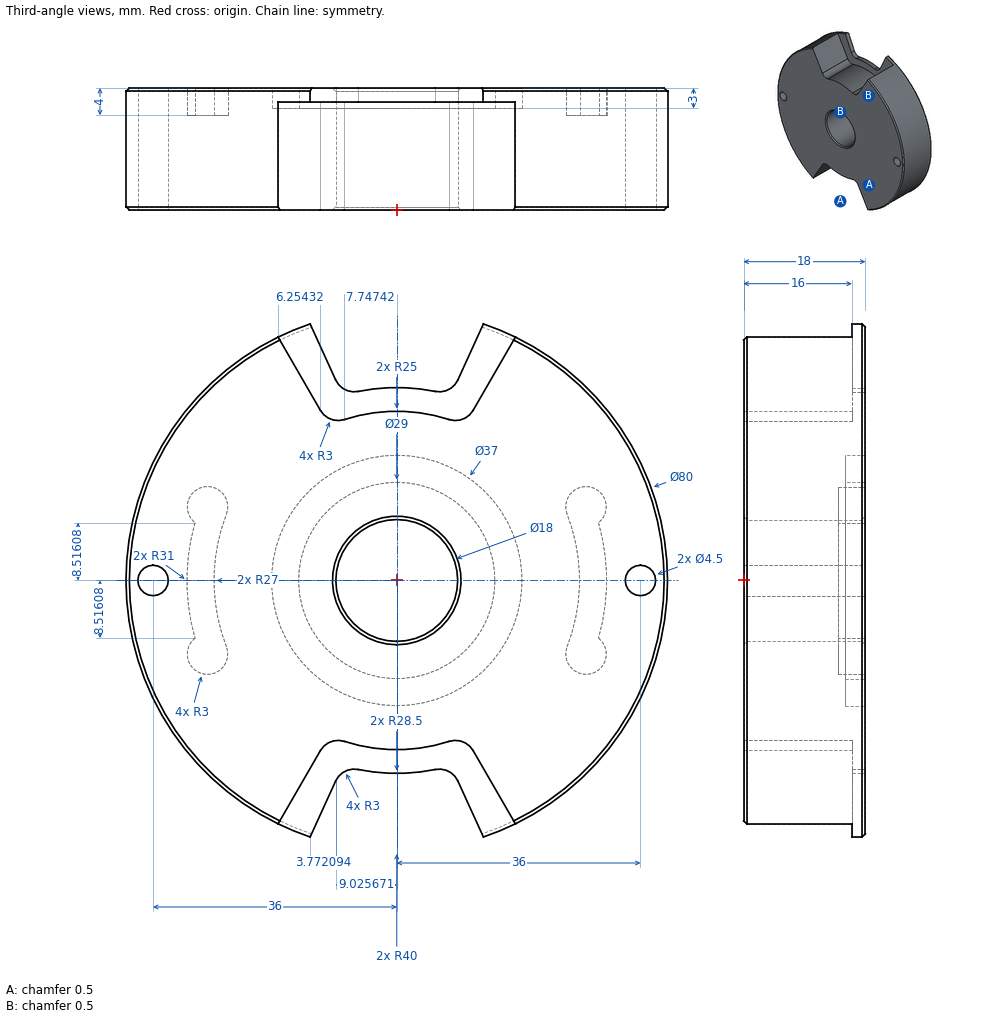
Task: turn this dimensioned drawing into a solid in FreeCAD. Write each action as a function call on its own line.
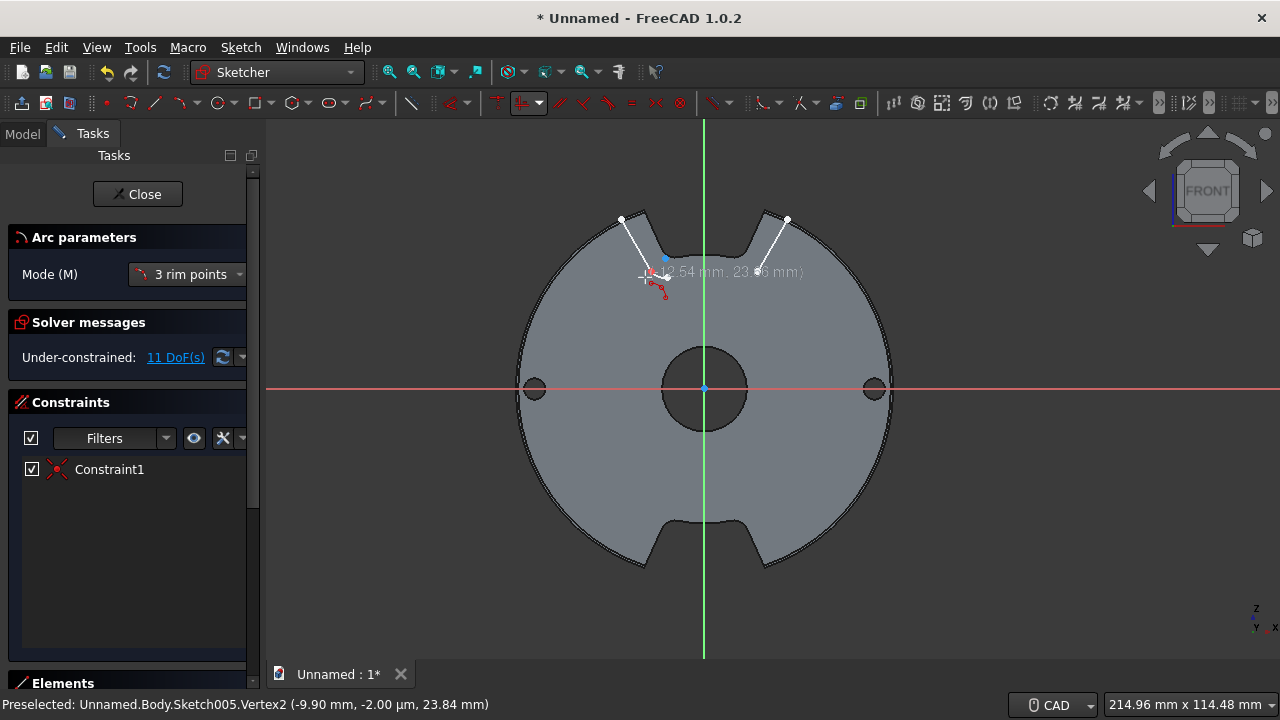
click(667, 278)
click(741, 277)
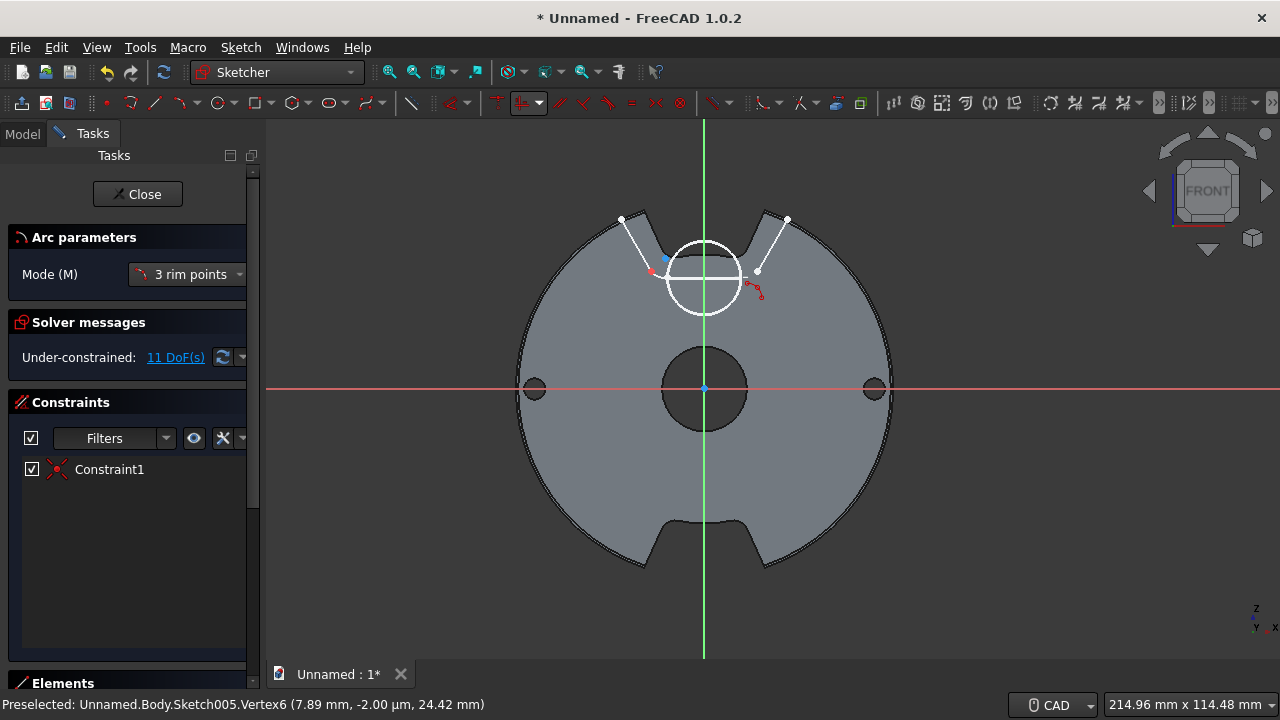
scroll(712, 271, up, 6)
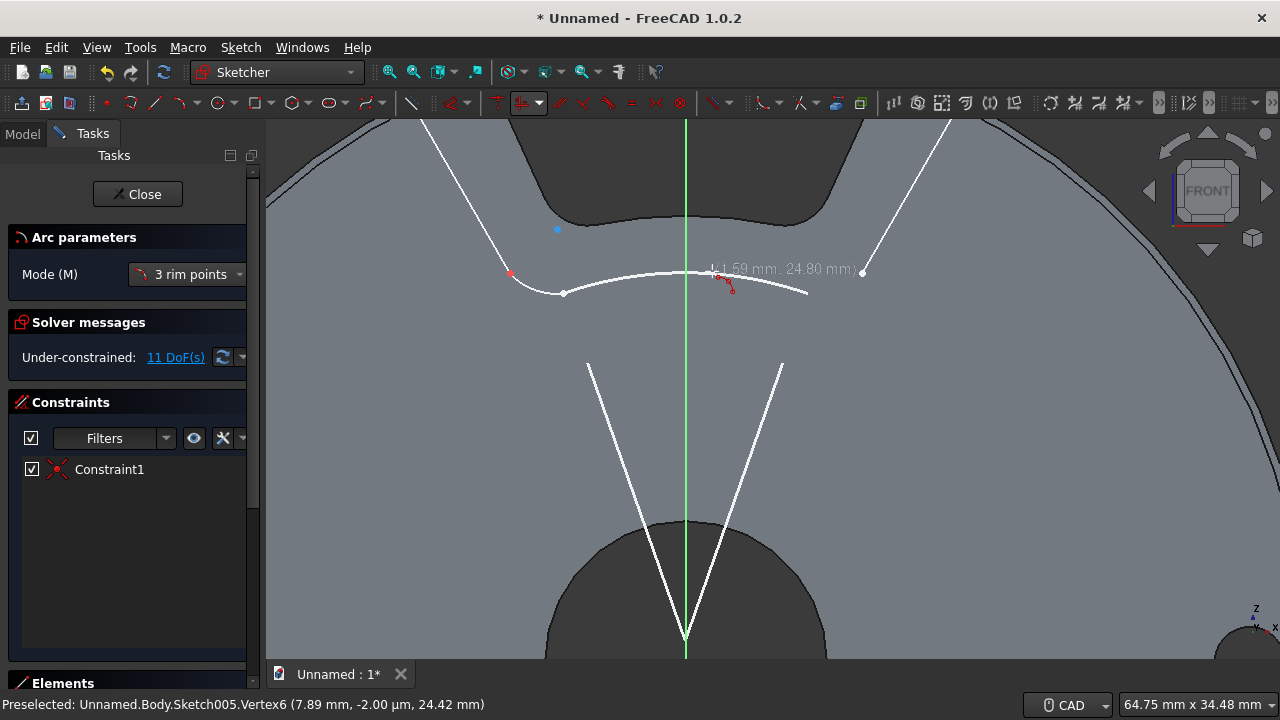
click(711, 271)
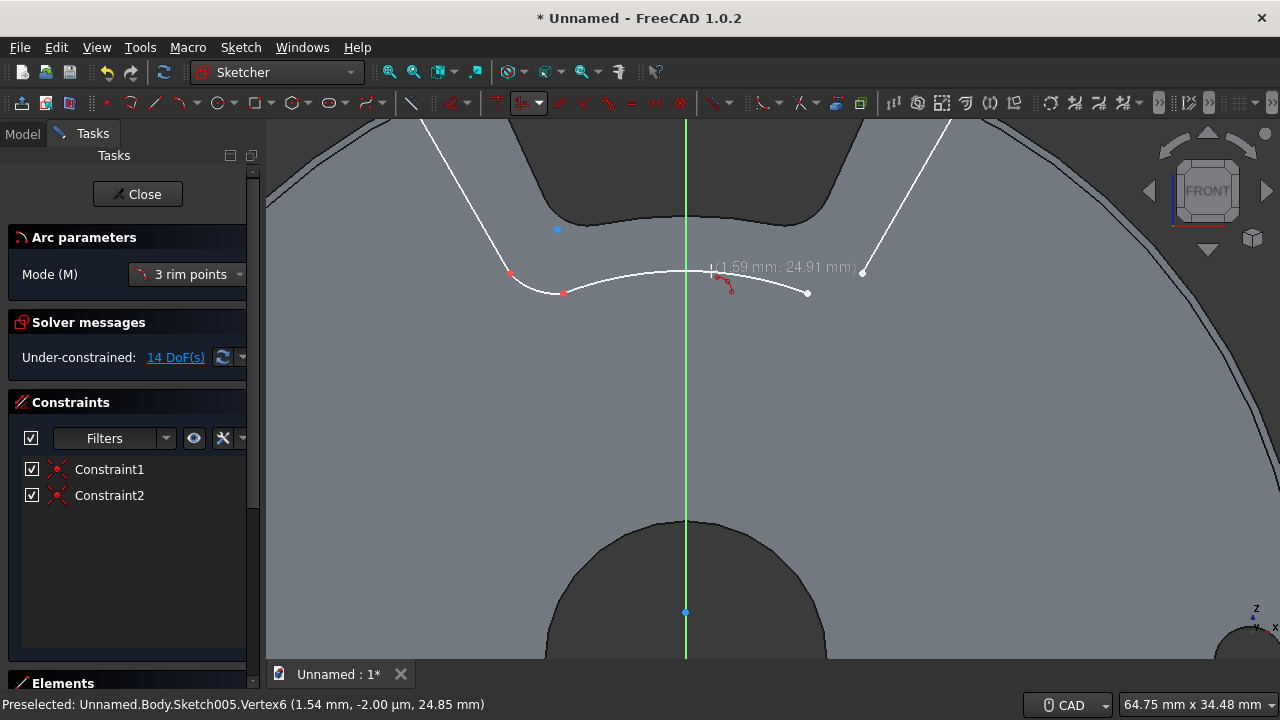
click(807, 294)
click(862, 274)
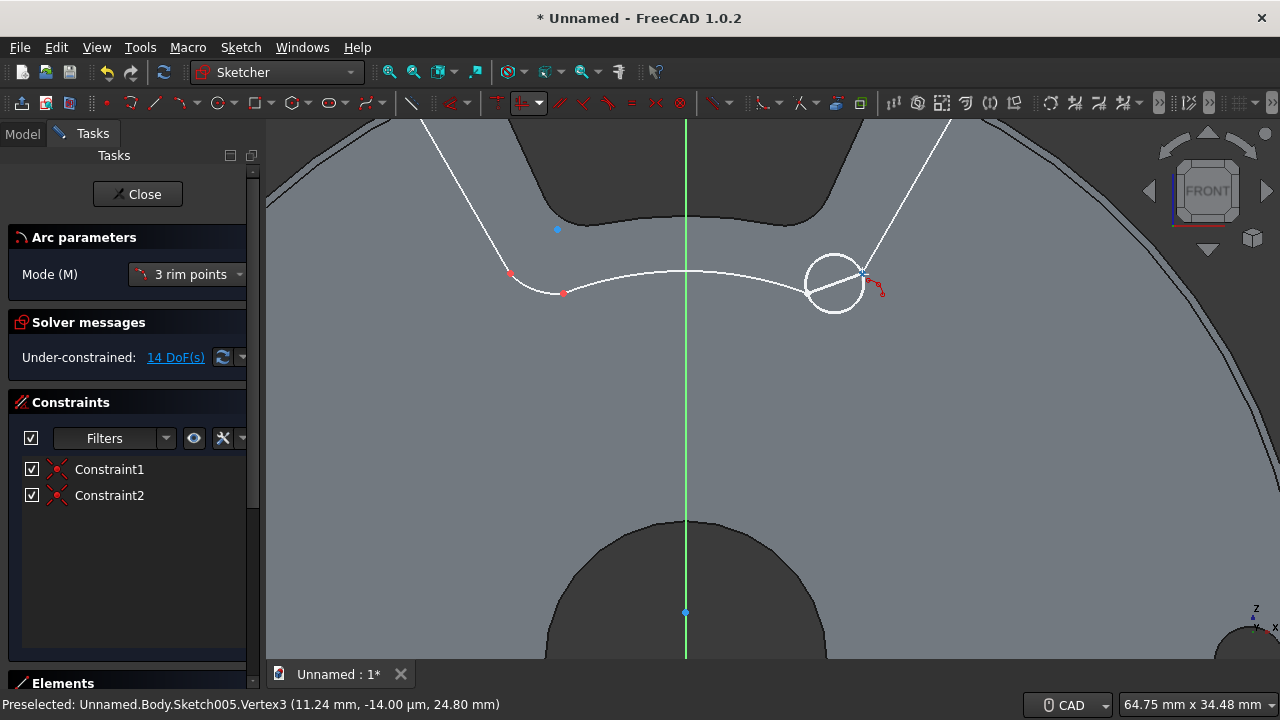
scroll(839, 289, up, 3)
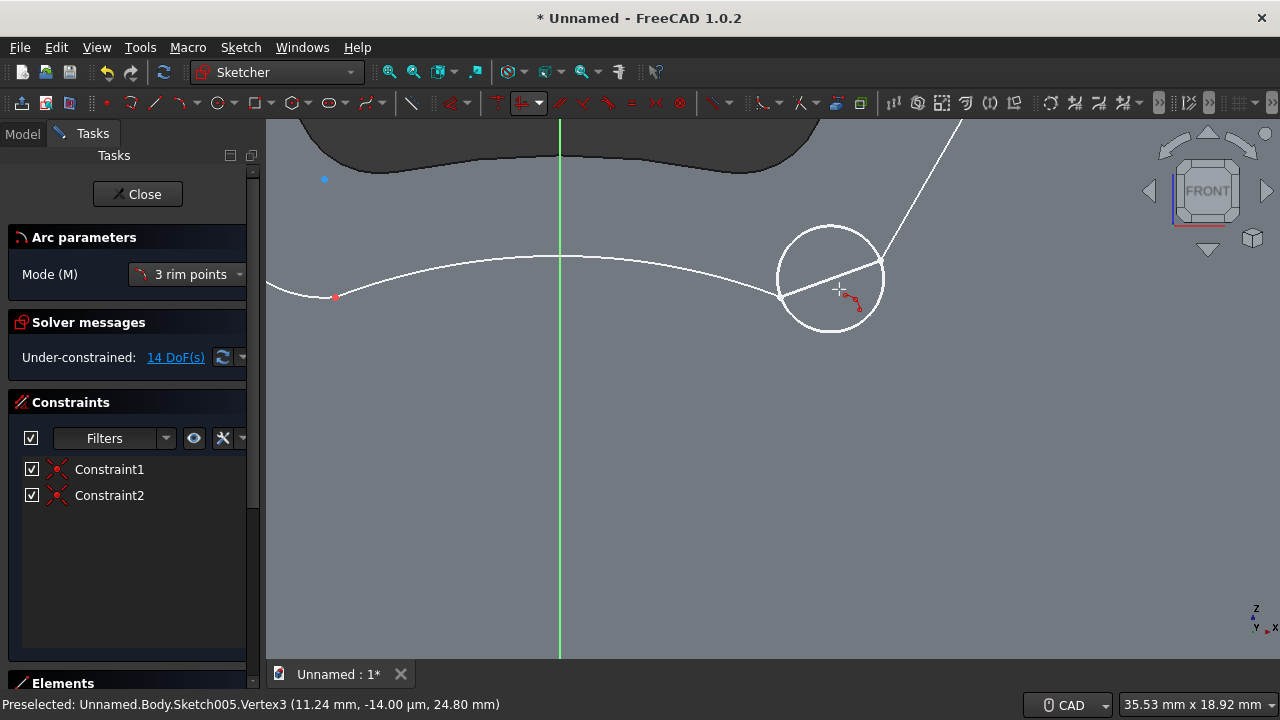
click(838, 289)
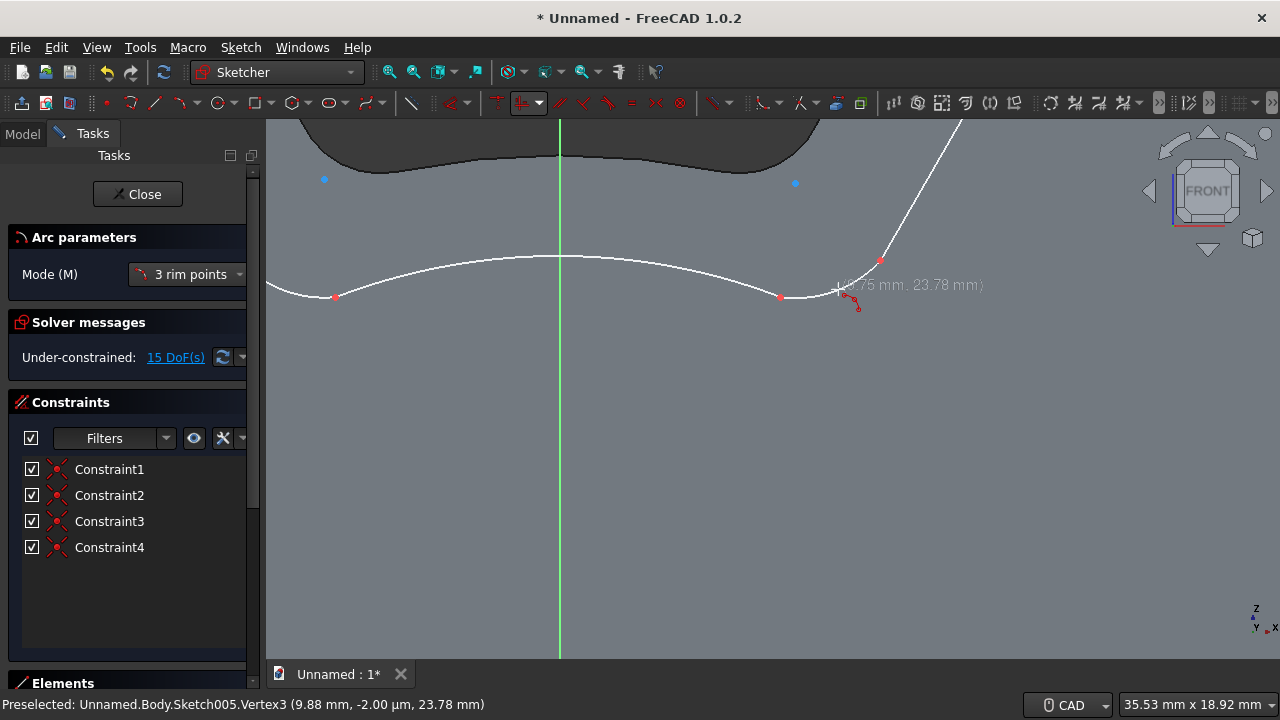
scroll(733, 274, down, 9)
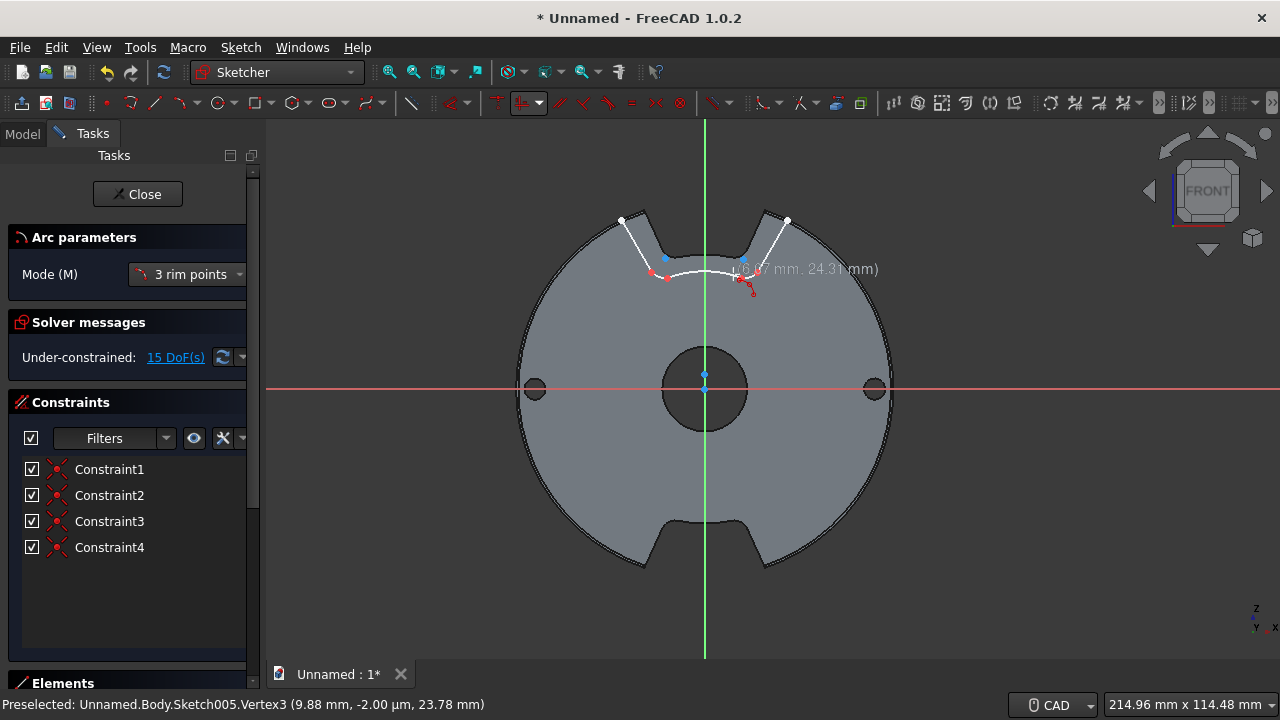
click(788, 220)
click(622, 220)
click(722, 201)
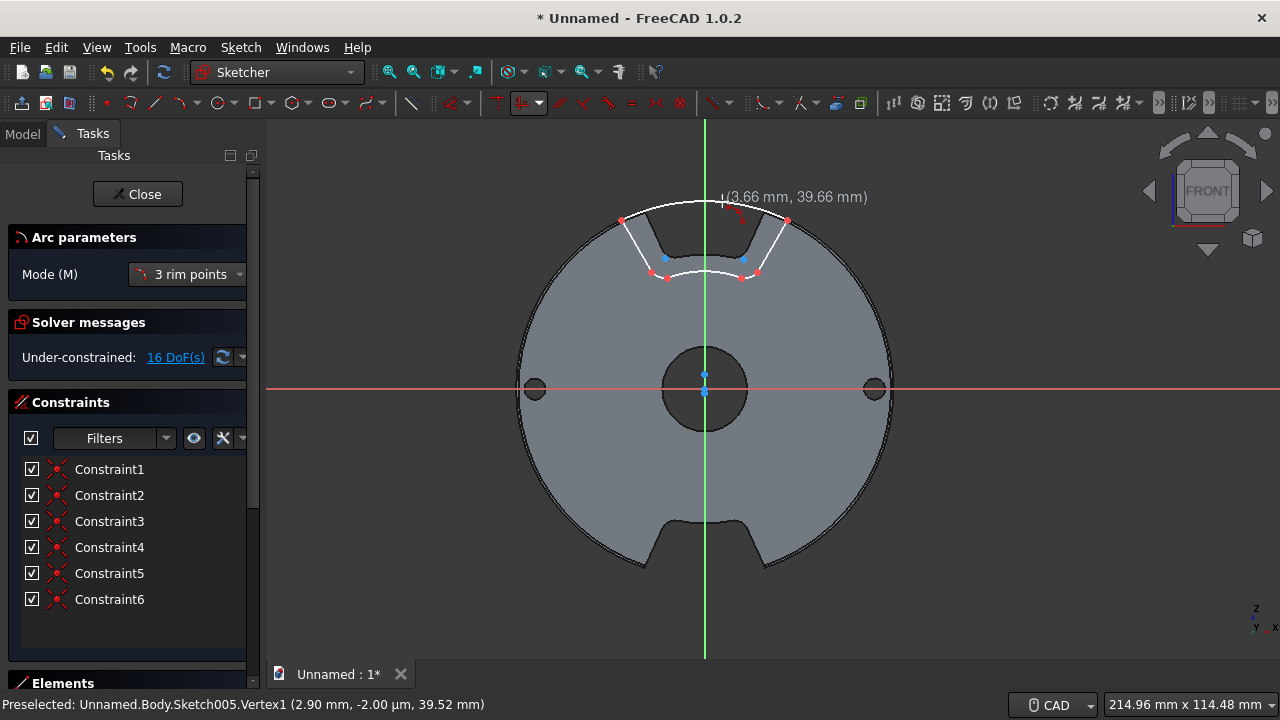
click(156, 104)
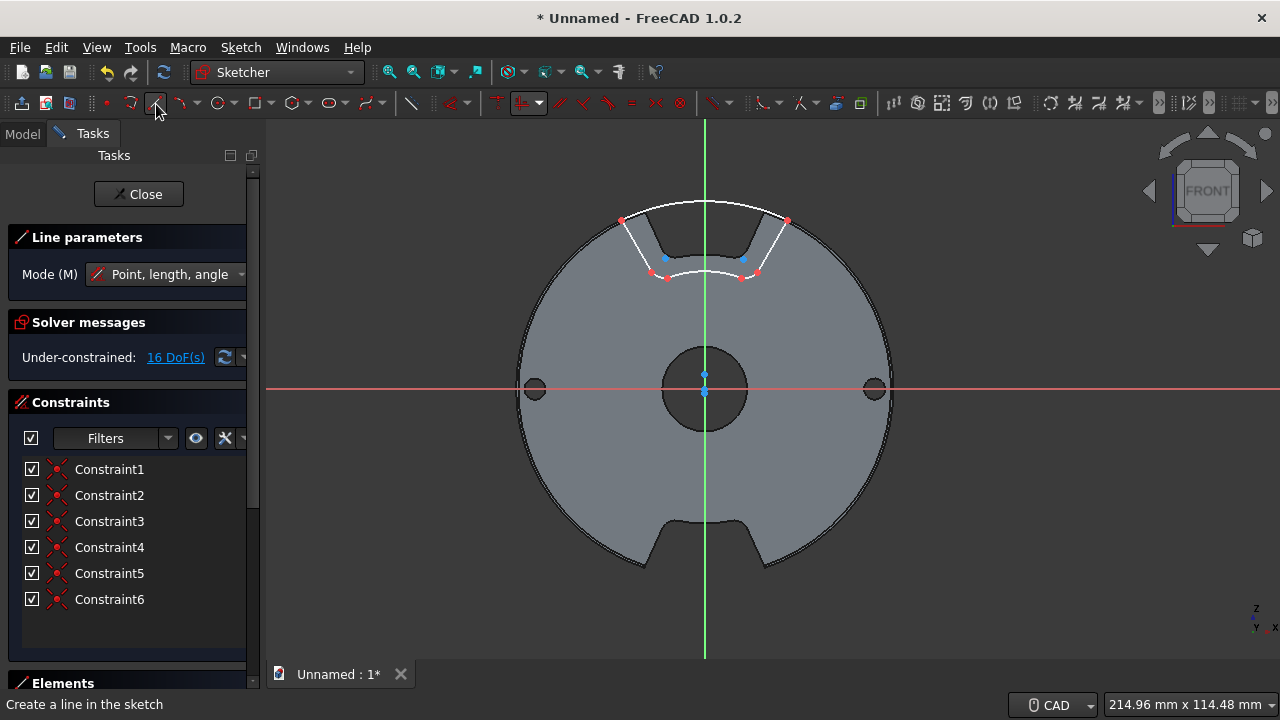
click(787, 559)
click(758, 508)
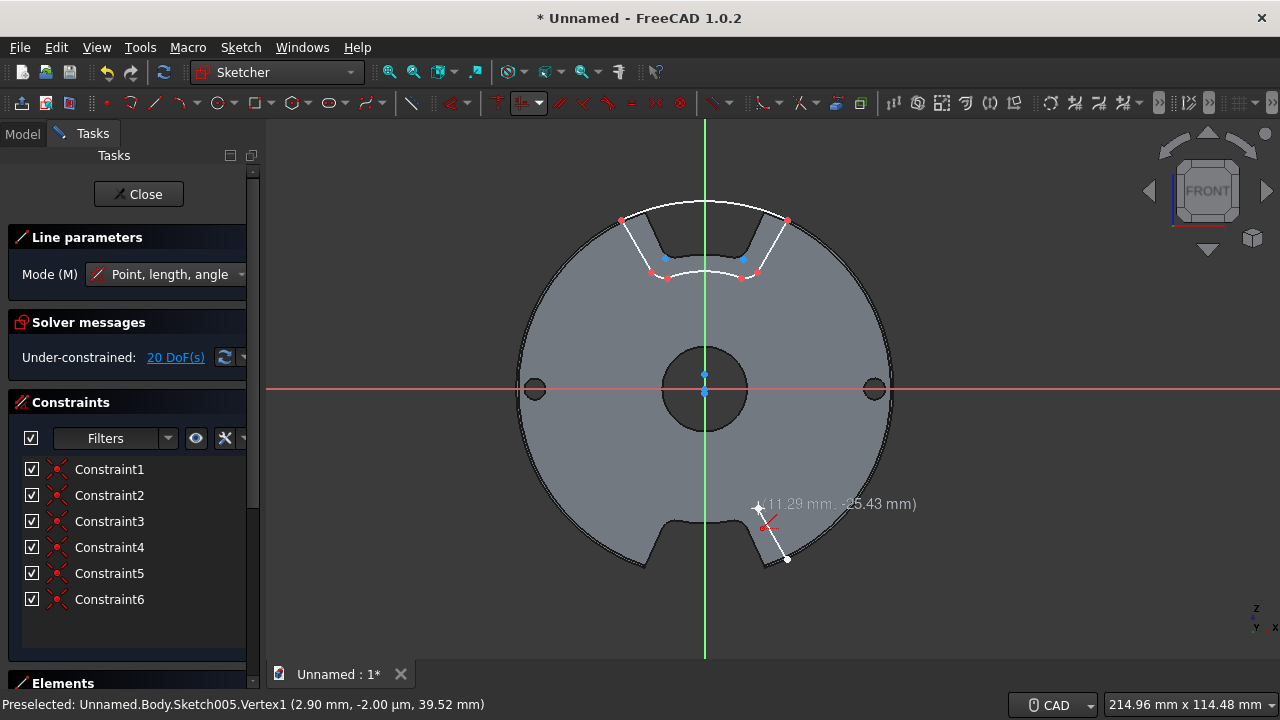
click(652, 508)
click(622, 559)